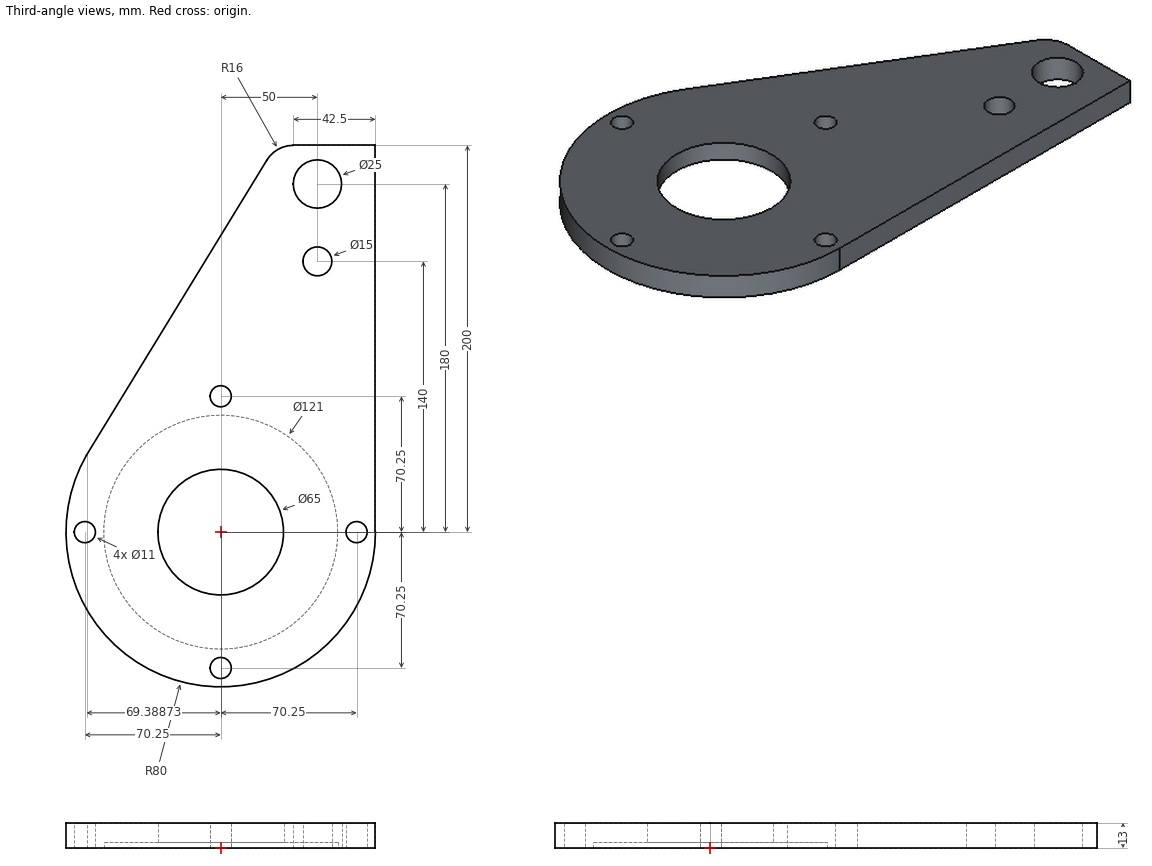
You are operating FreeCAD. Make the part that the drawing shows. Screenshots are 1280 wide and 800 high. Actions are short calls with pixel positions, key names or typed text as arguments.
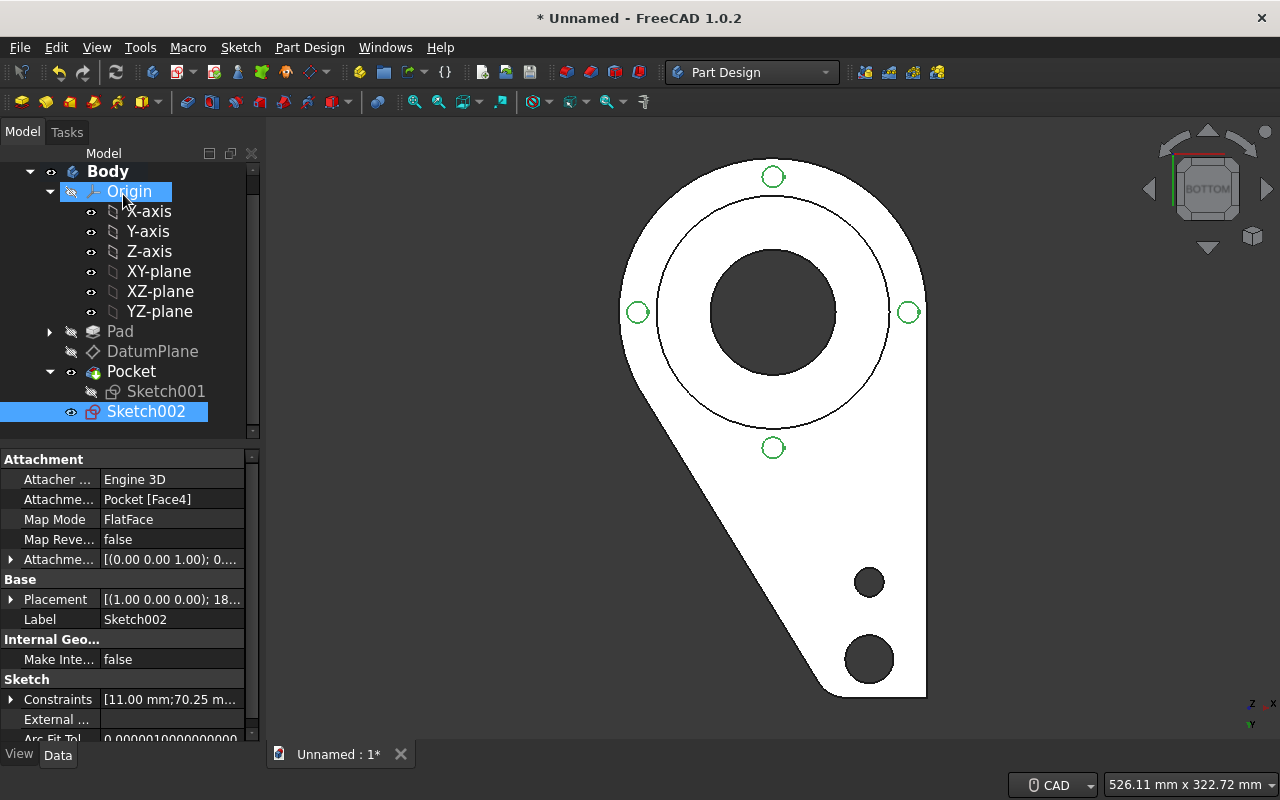
click(188, 102)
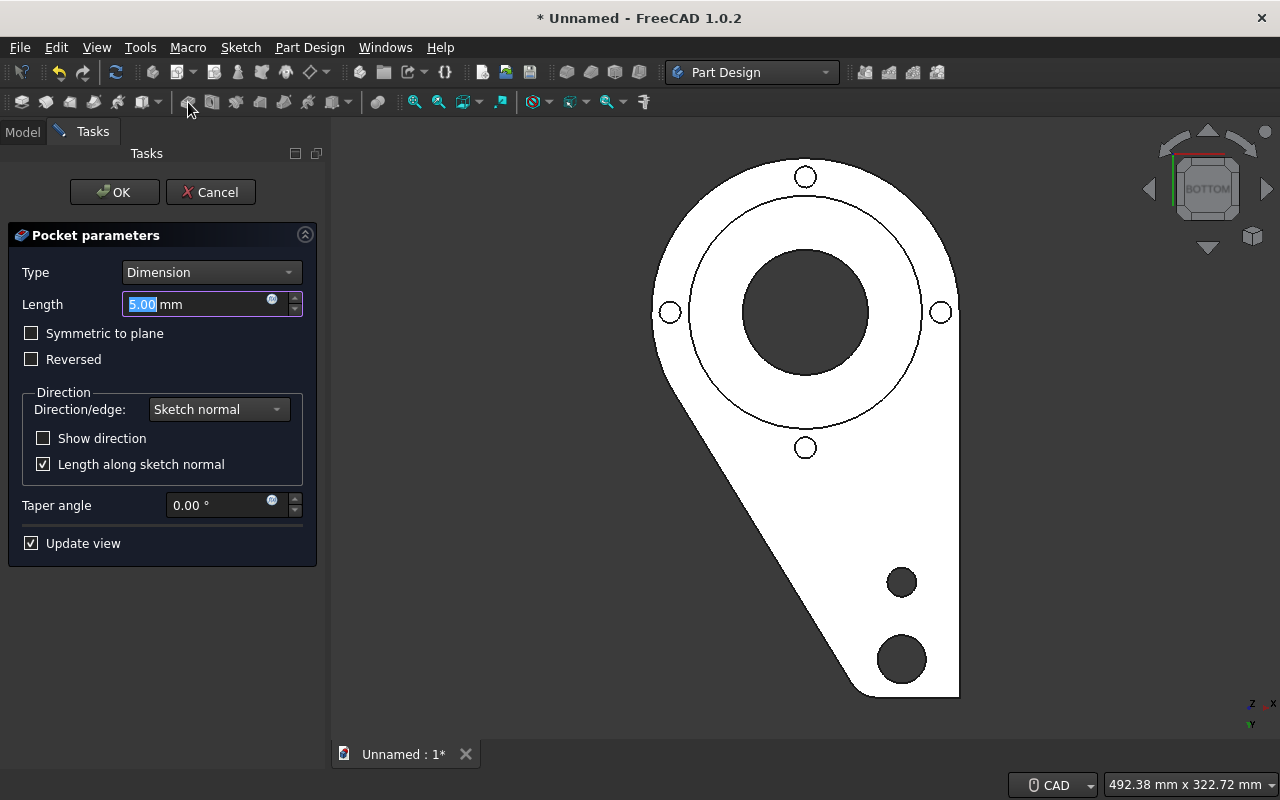
click(212, 272)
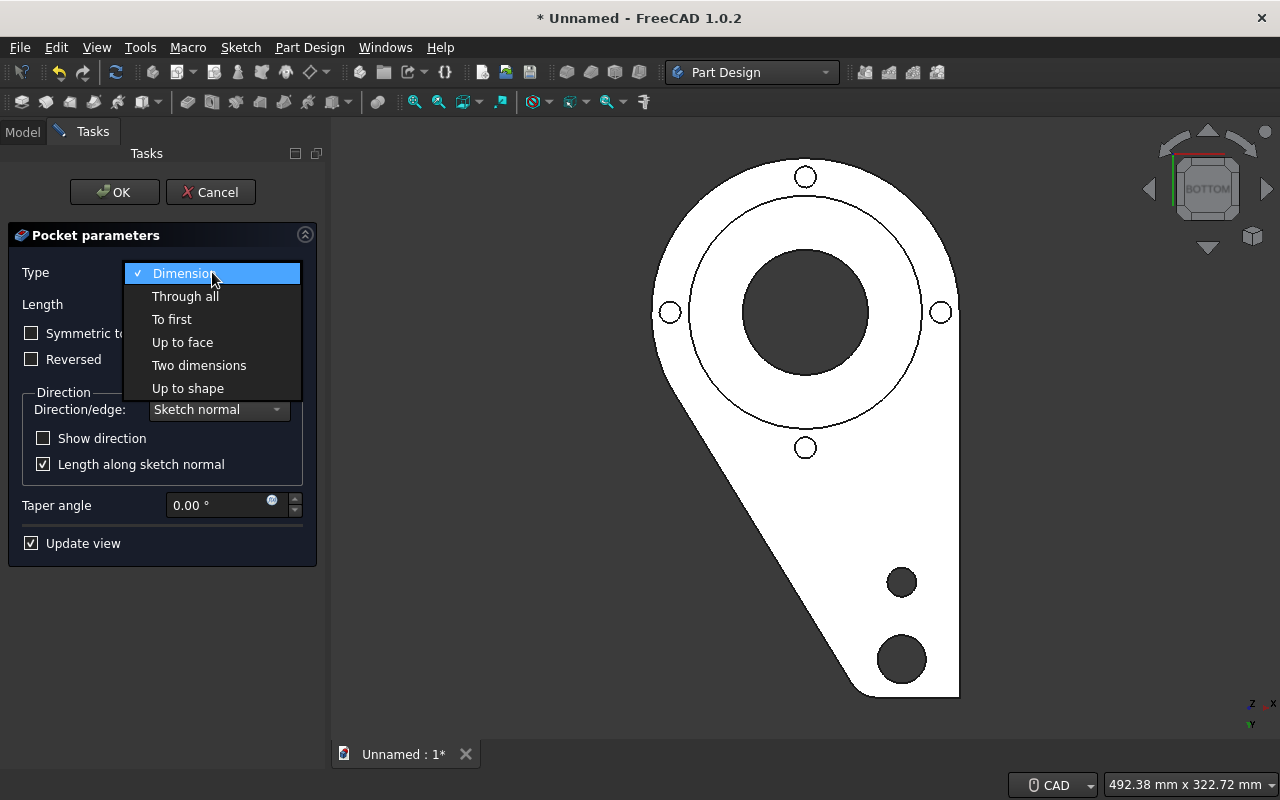
click(212, 296)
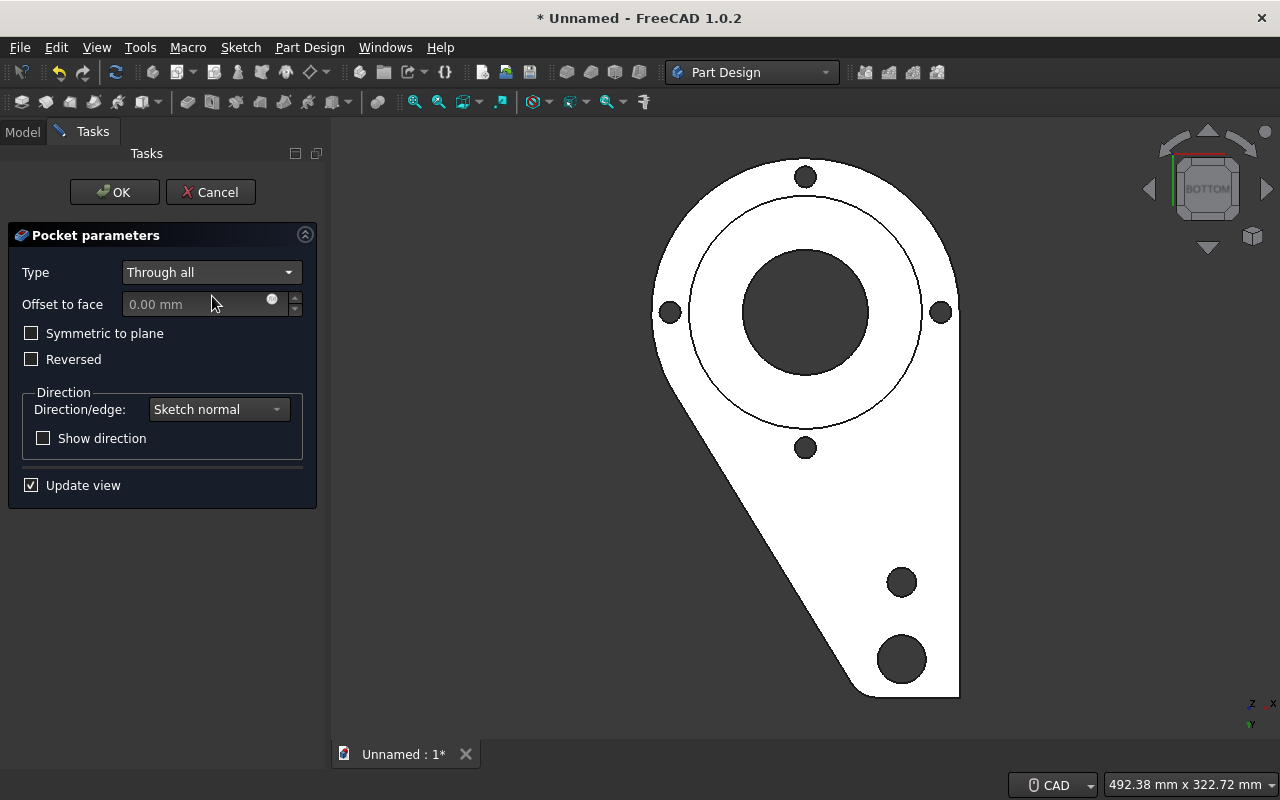
click(115, 192)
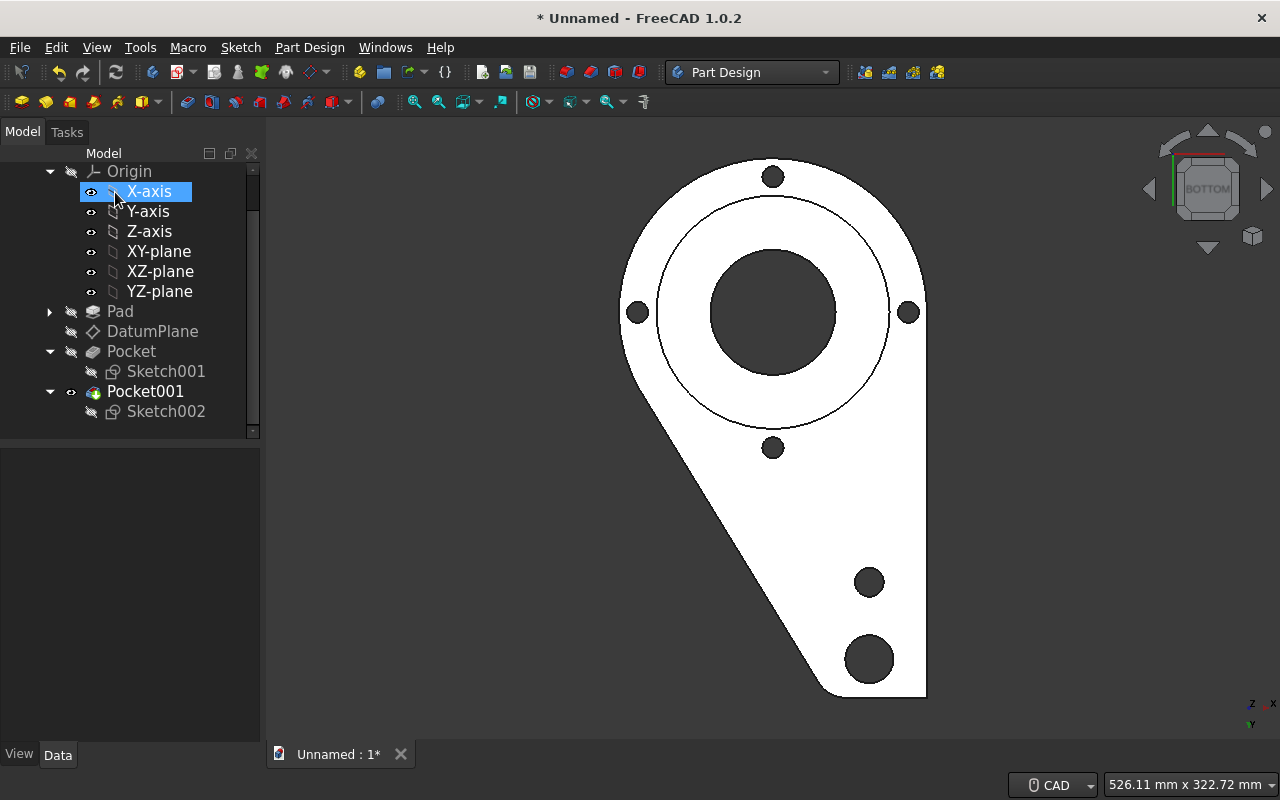
key(0)